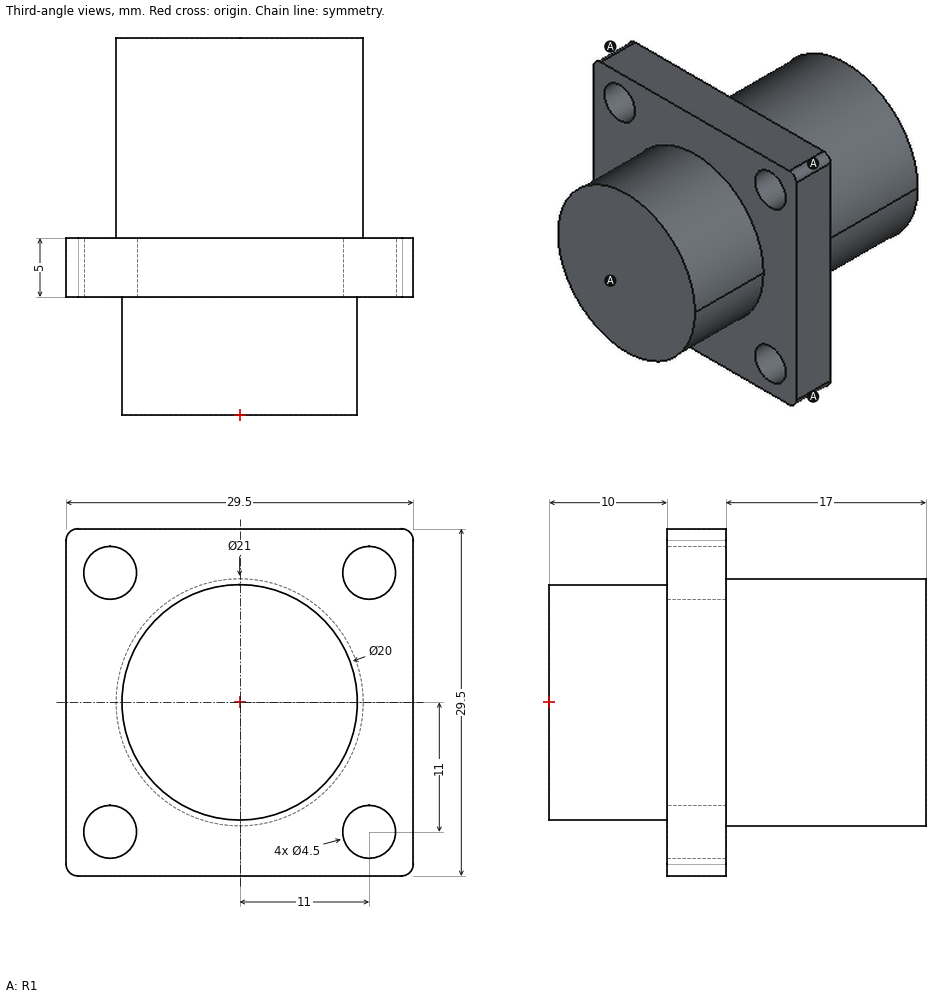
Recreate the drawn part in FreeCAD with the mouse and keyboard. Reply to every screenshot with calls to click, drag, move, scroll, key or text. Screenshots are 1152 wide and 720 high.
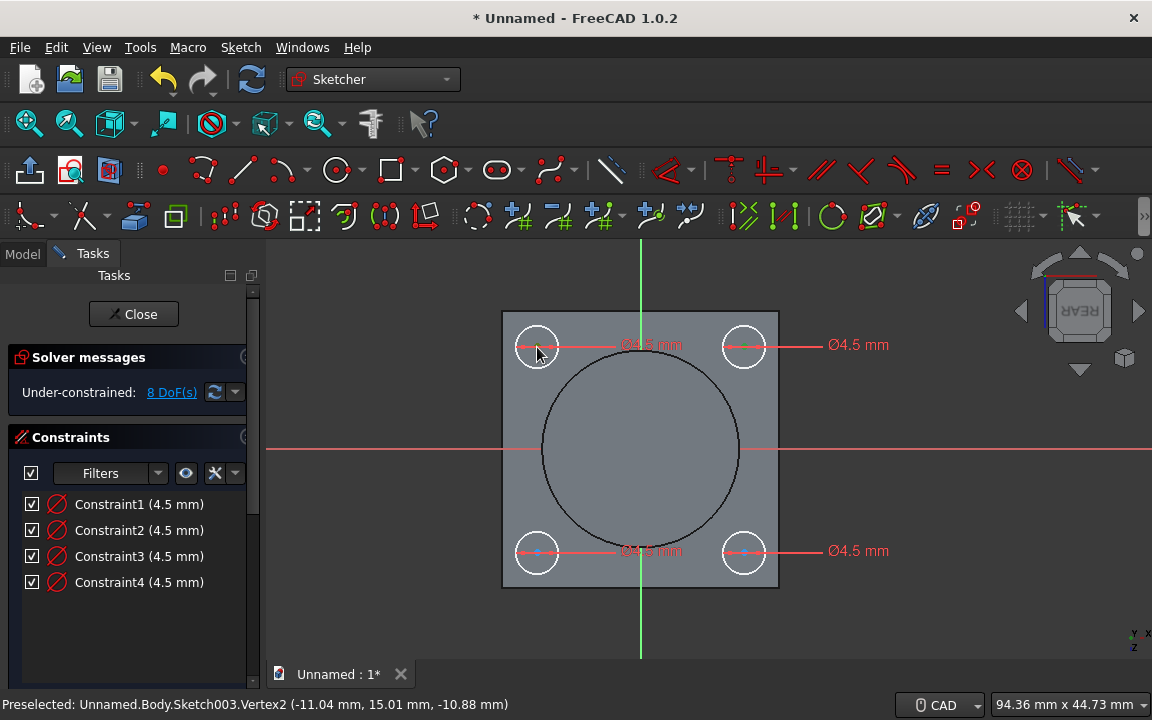
click(641, 605)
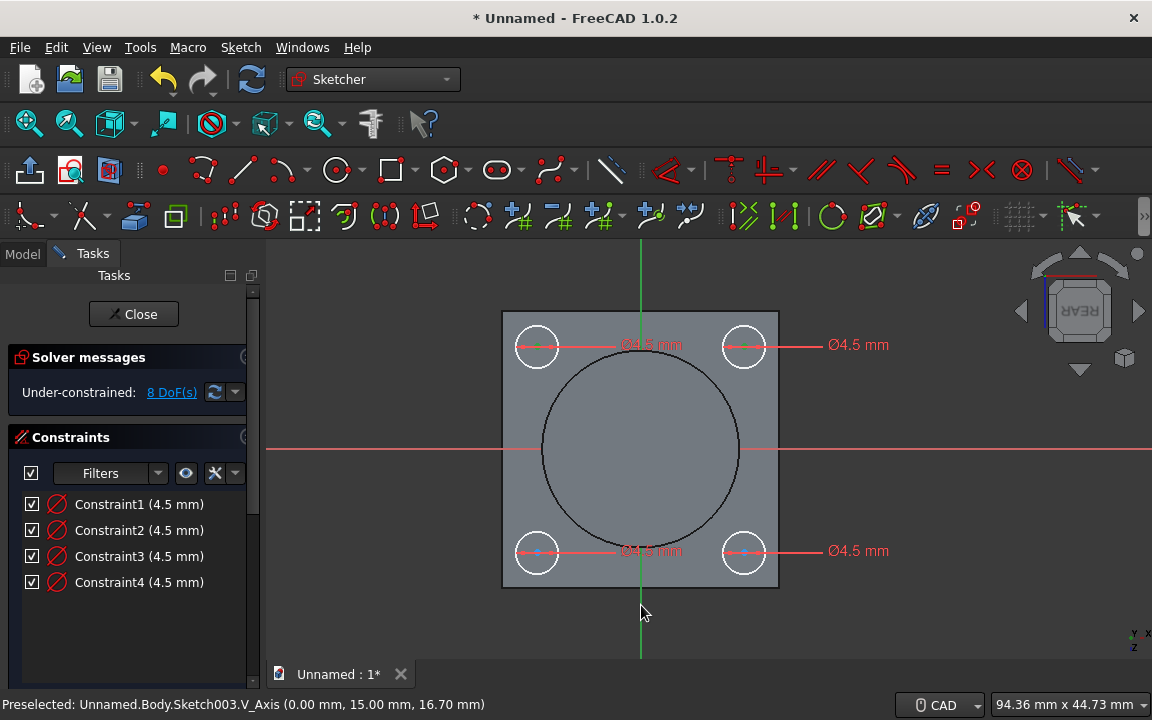
key(s)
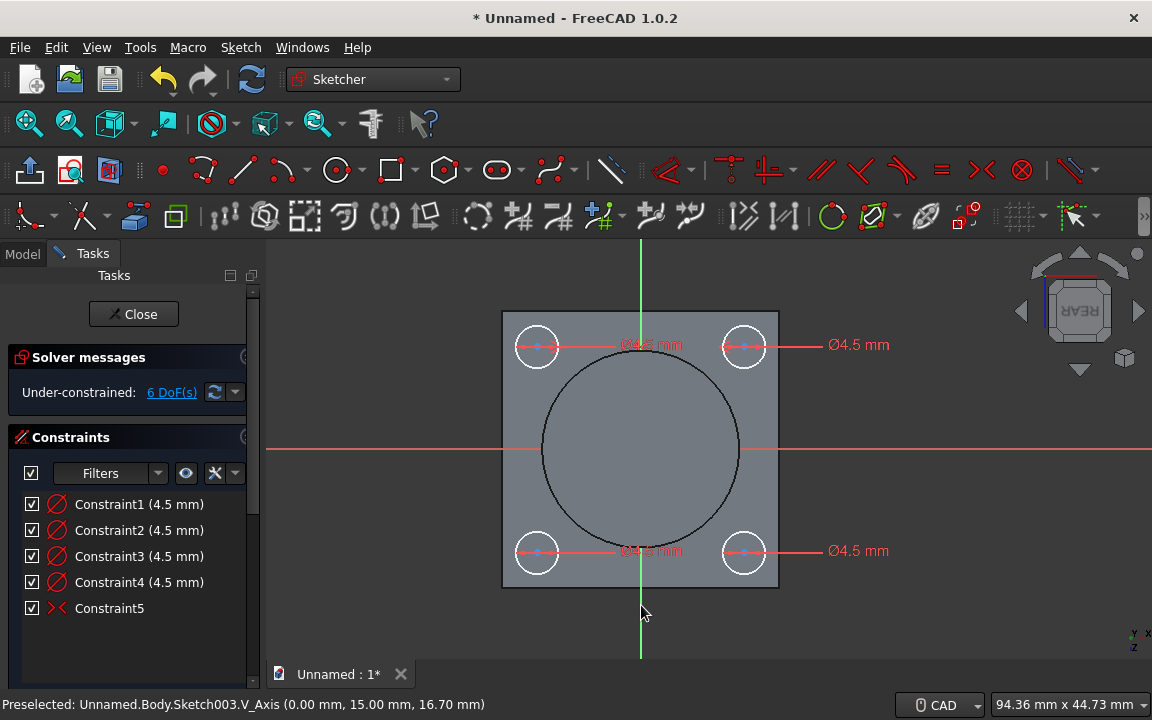
click(537, 347)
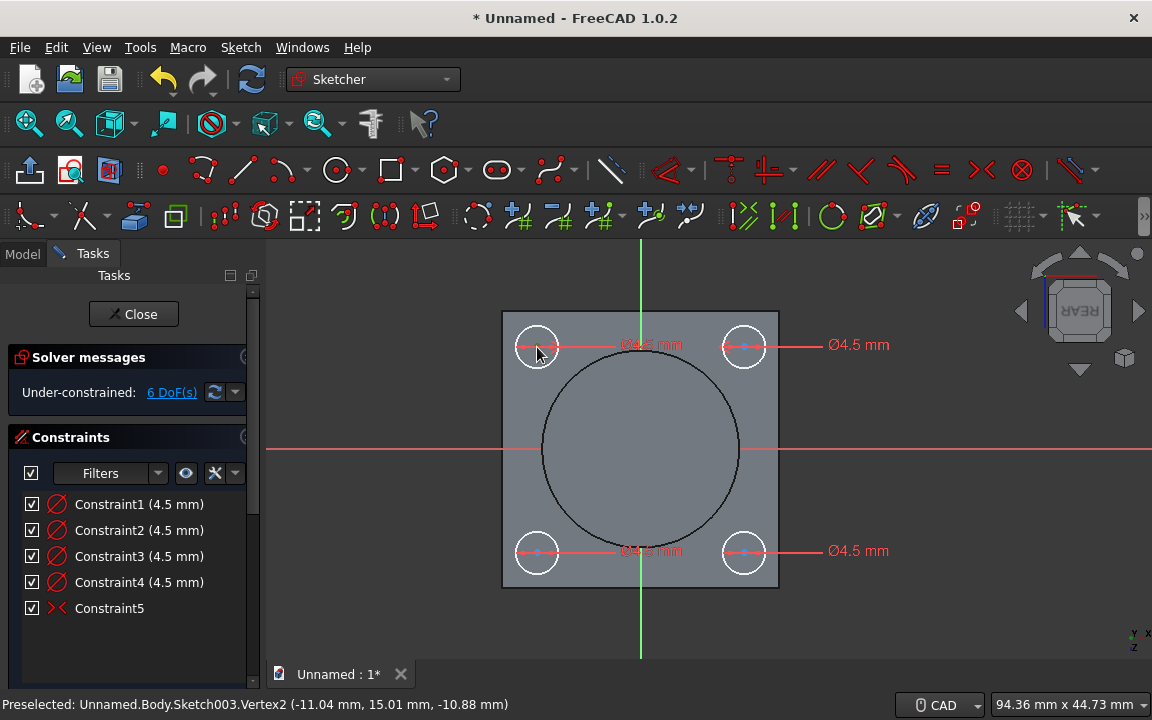
click(537, 553)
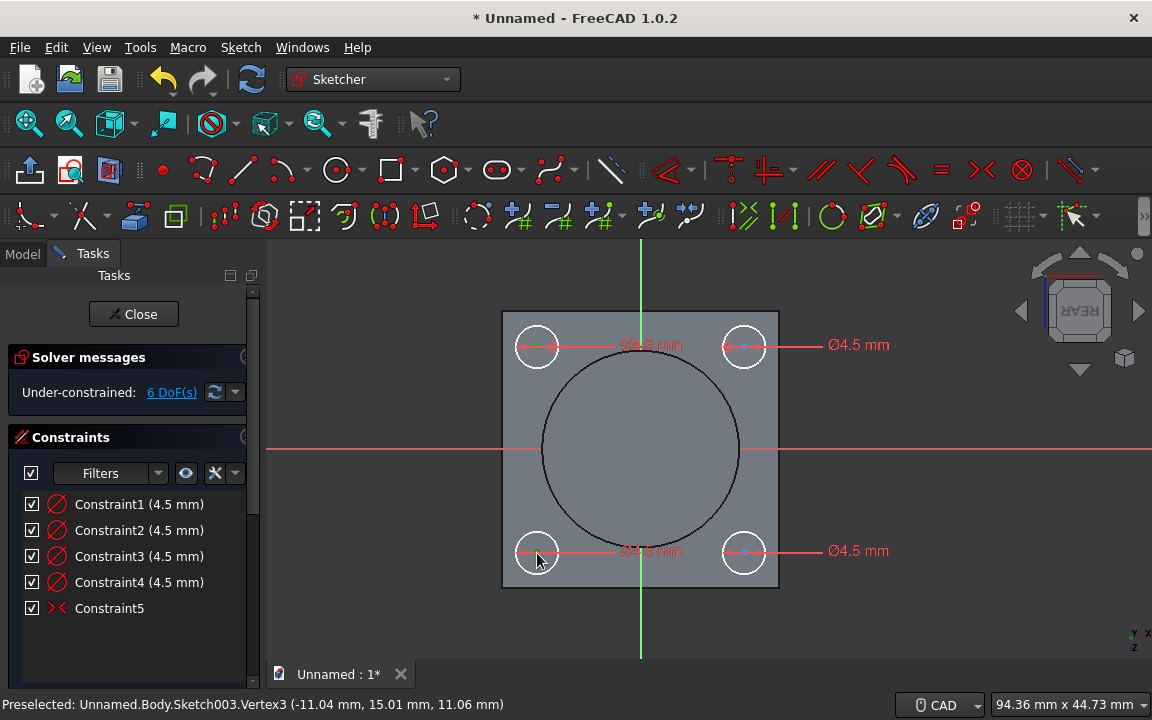
click(344, 449)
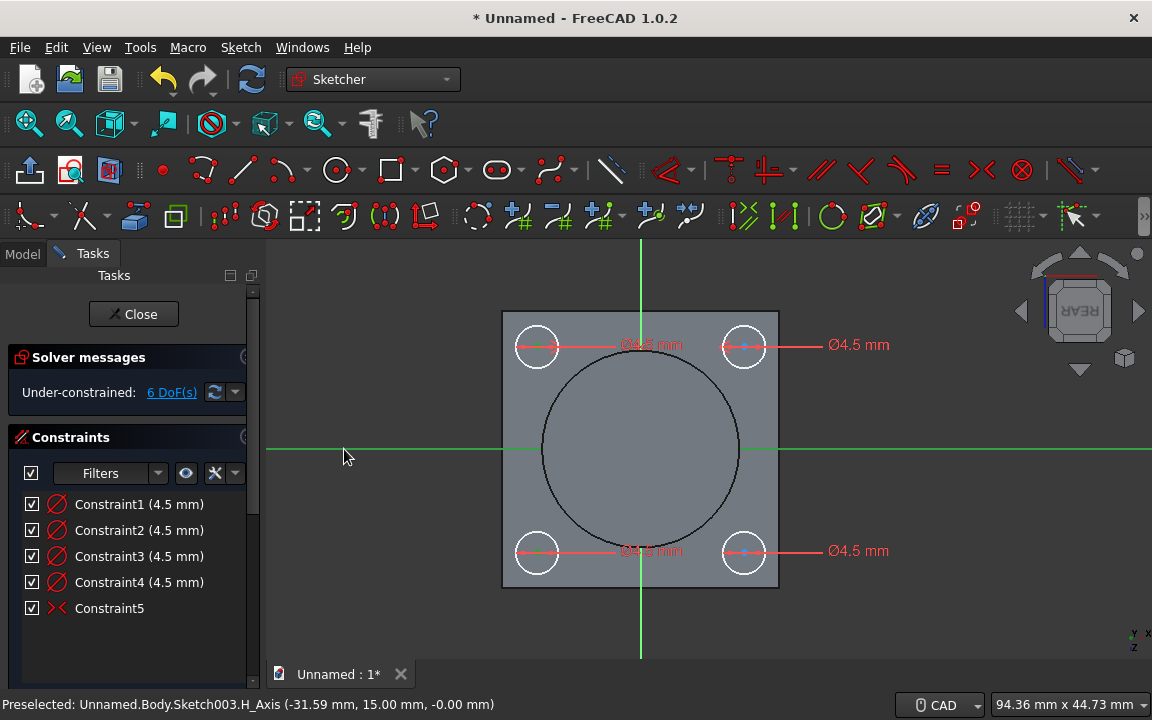
click(982, 170)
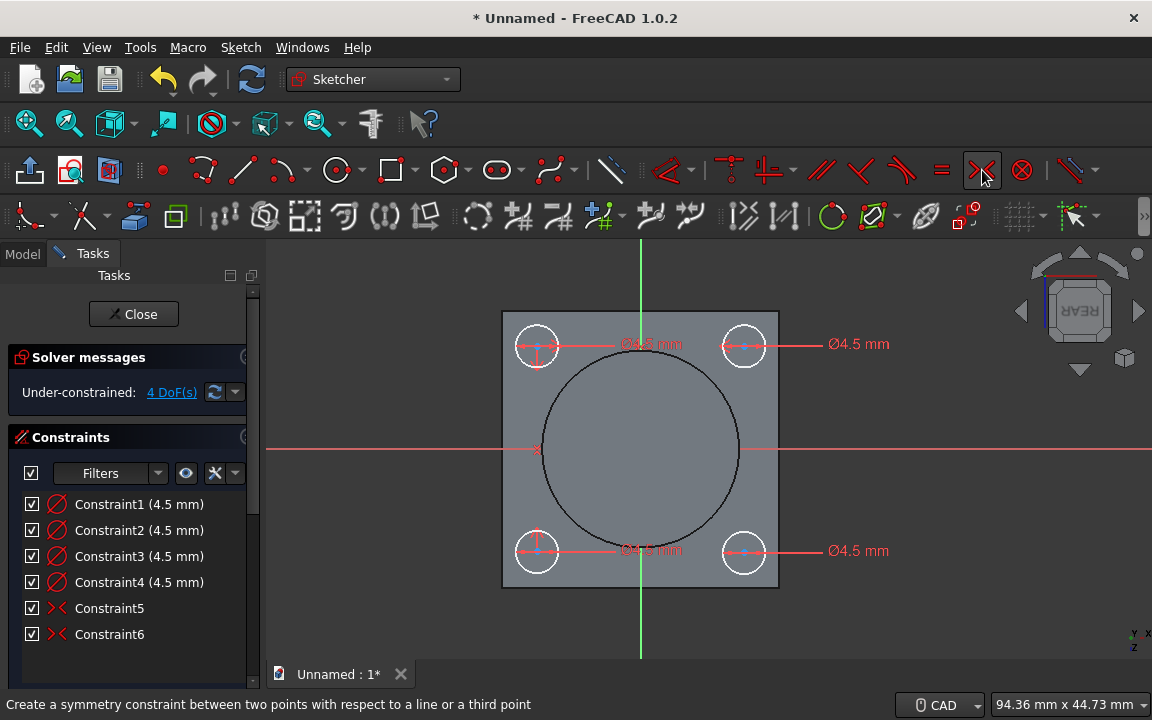
click(744, 346)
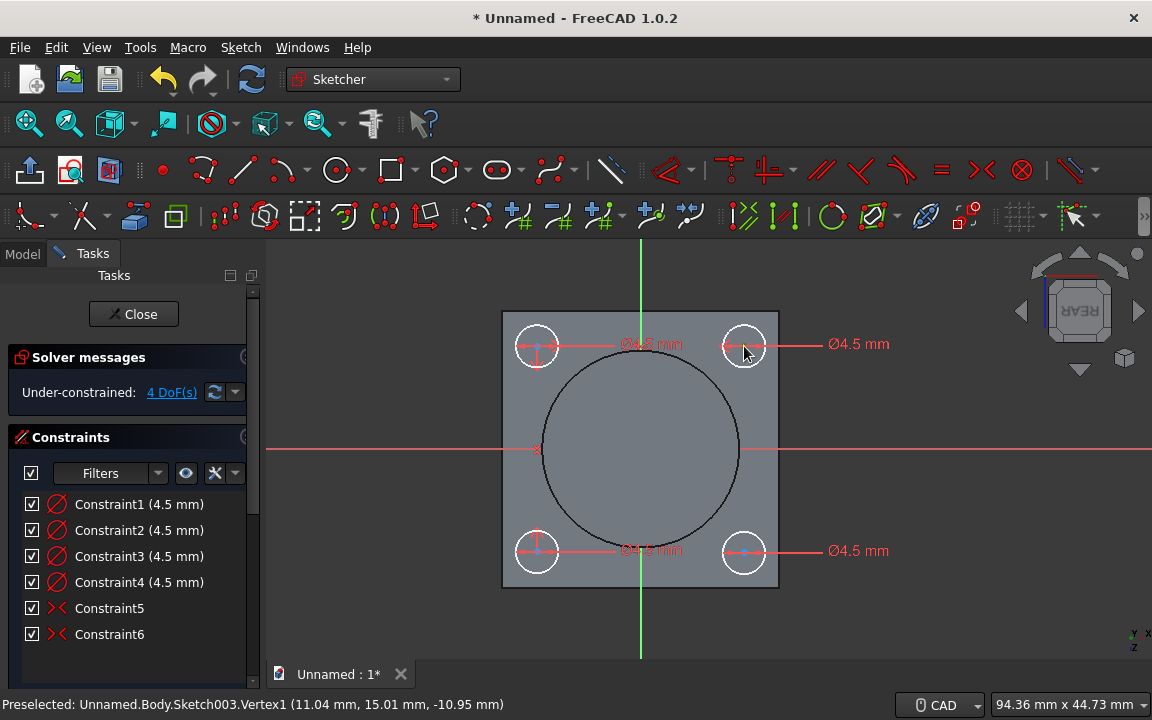
click(744, 553)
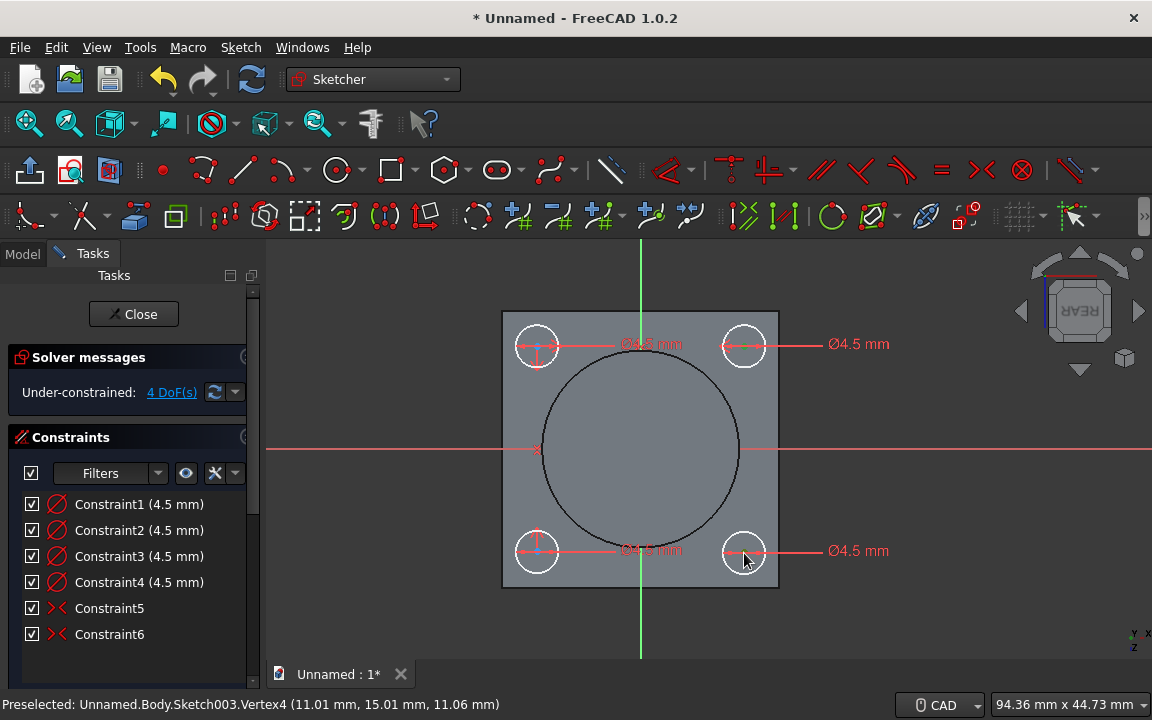
click(344, 449)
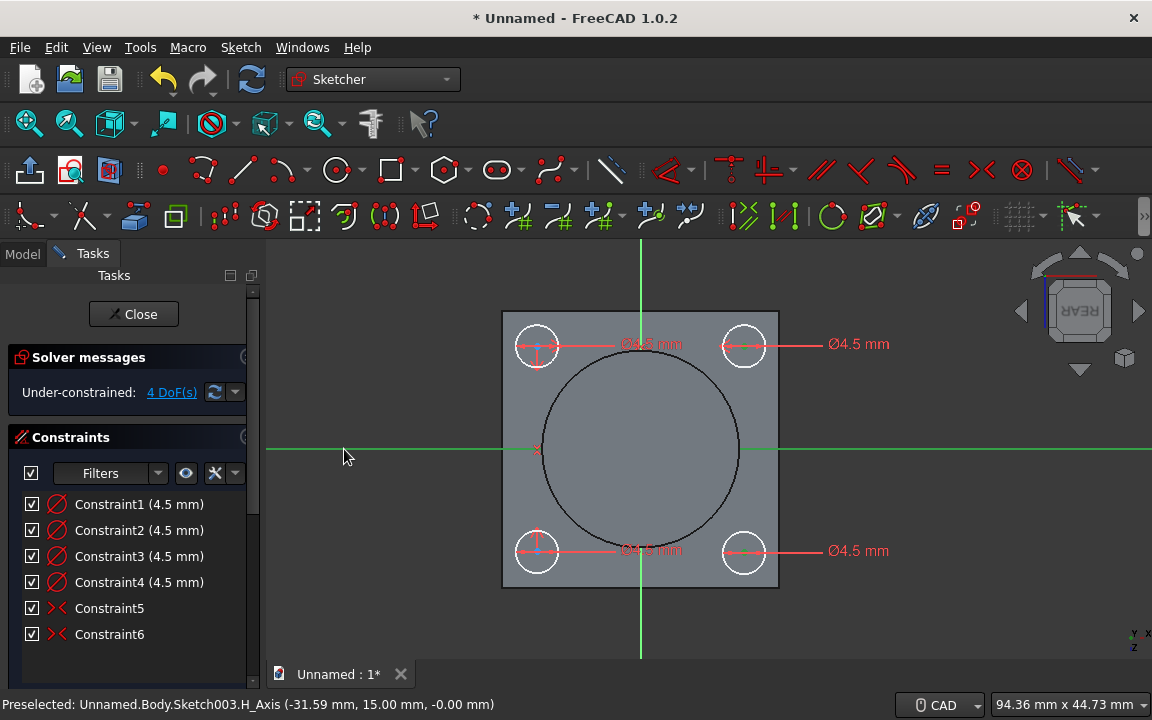
click(982, 170)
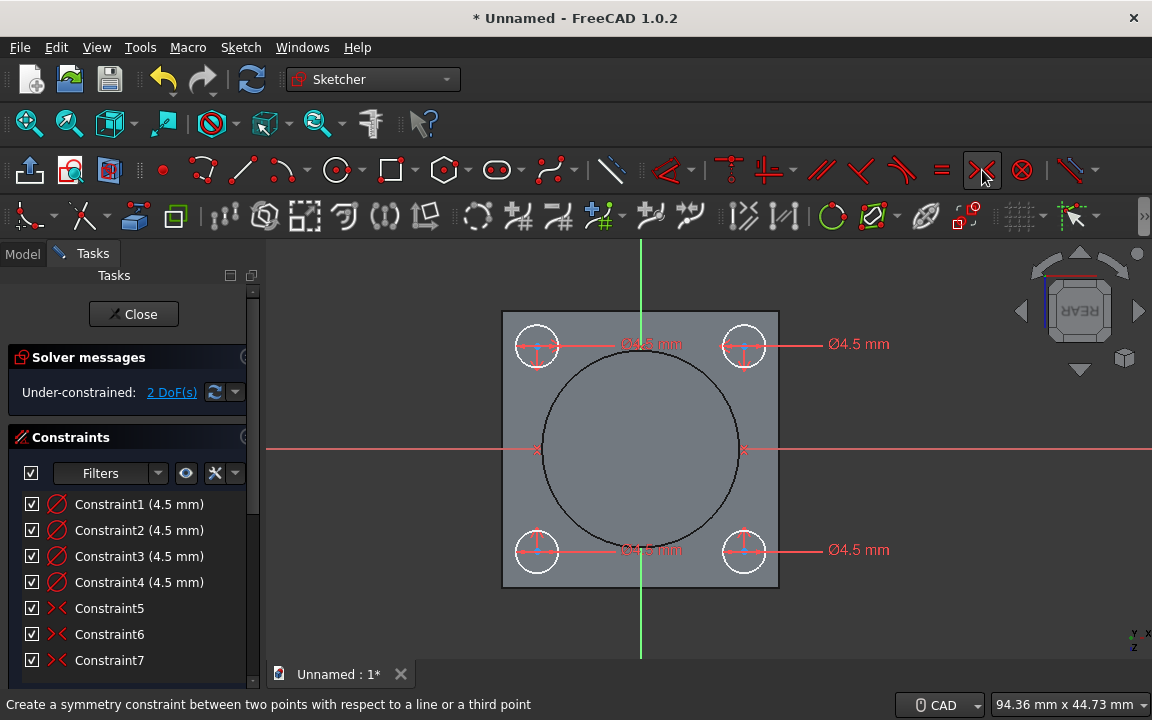
key(d)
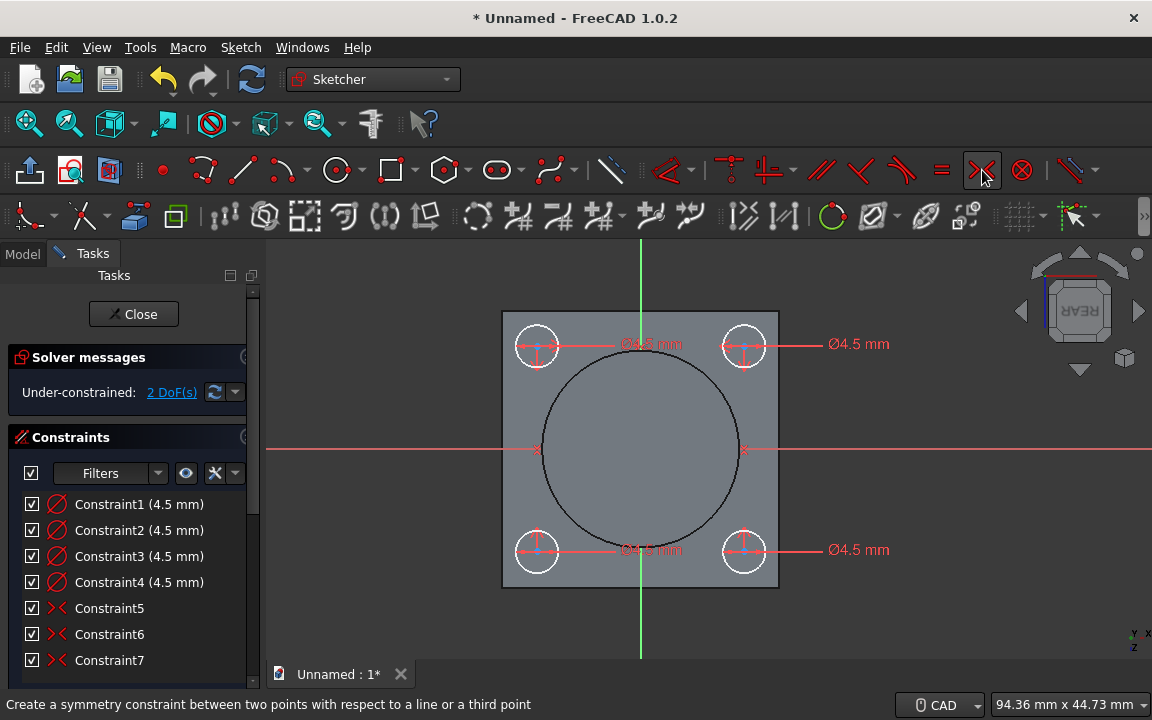
click(744, 346)
click(692, 312)